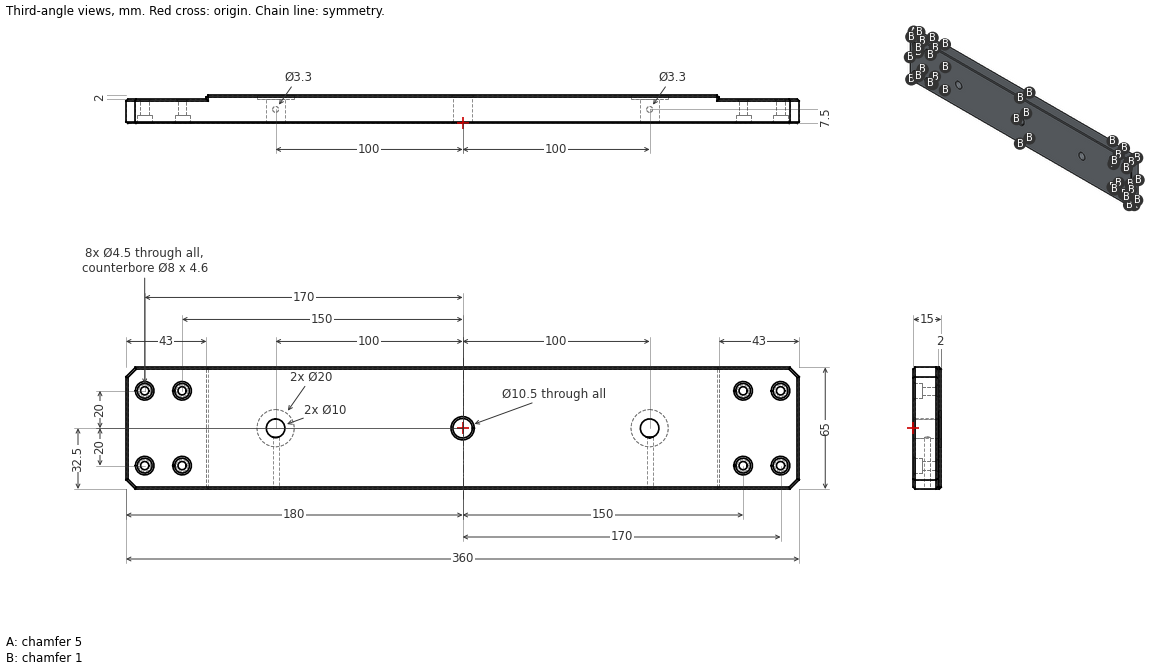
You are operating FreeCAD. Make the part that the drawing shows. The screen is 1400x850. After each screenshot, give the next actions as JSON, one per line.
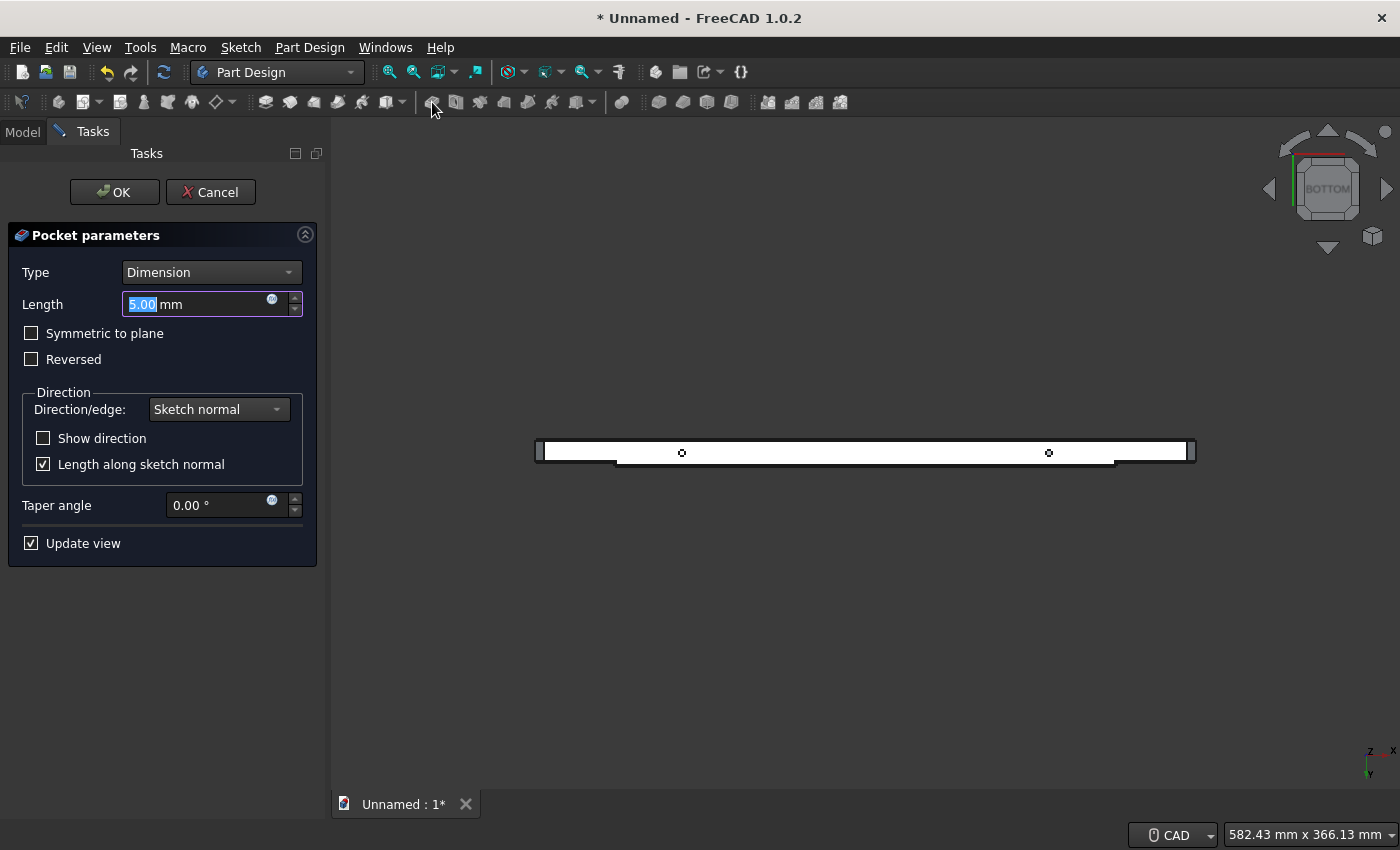
{"action": "left_click", "coordinate": [212, 272]}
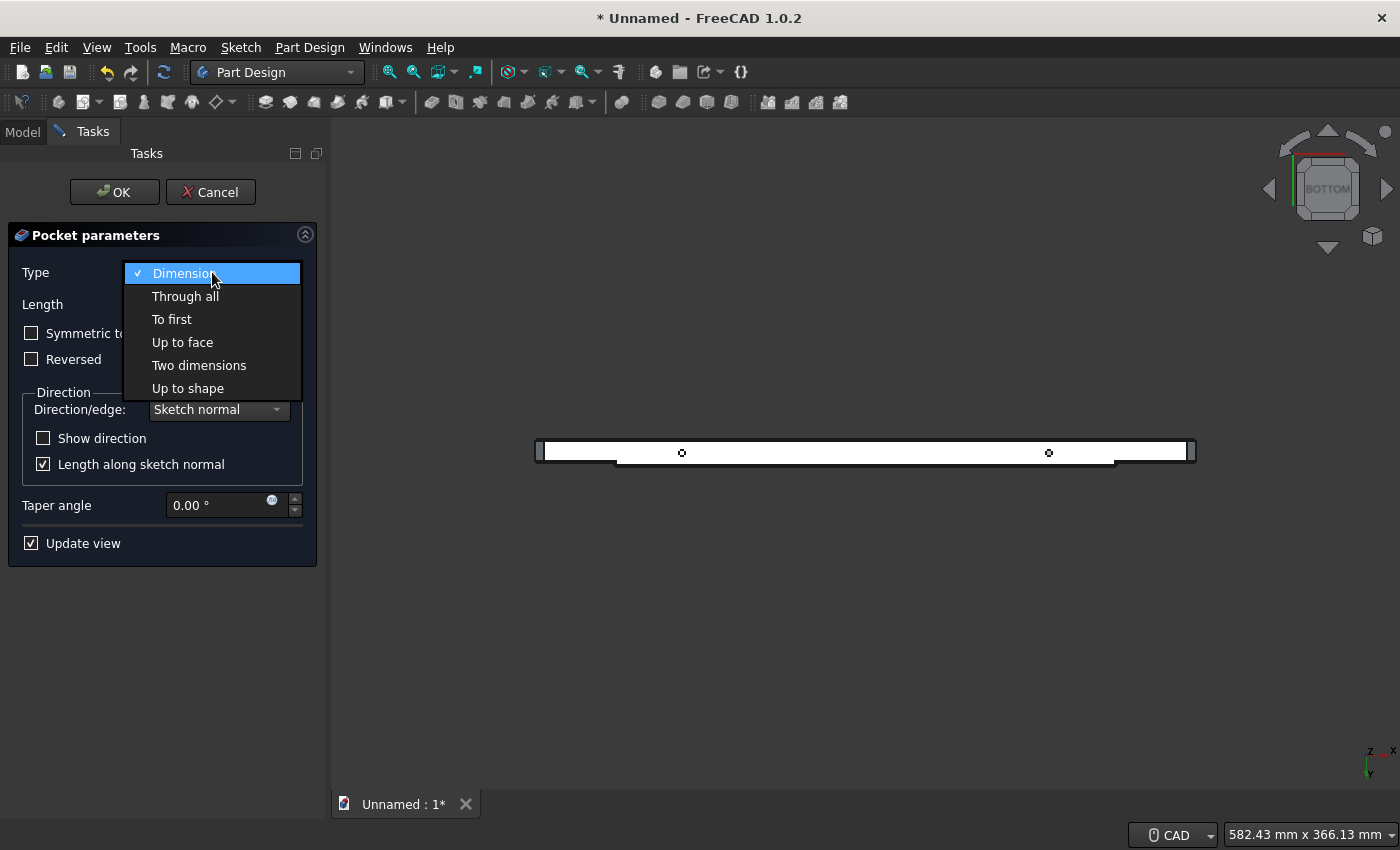
{"action": "left_click", "coordinate": [212, 320]}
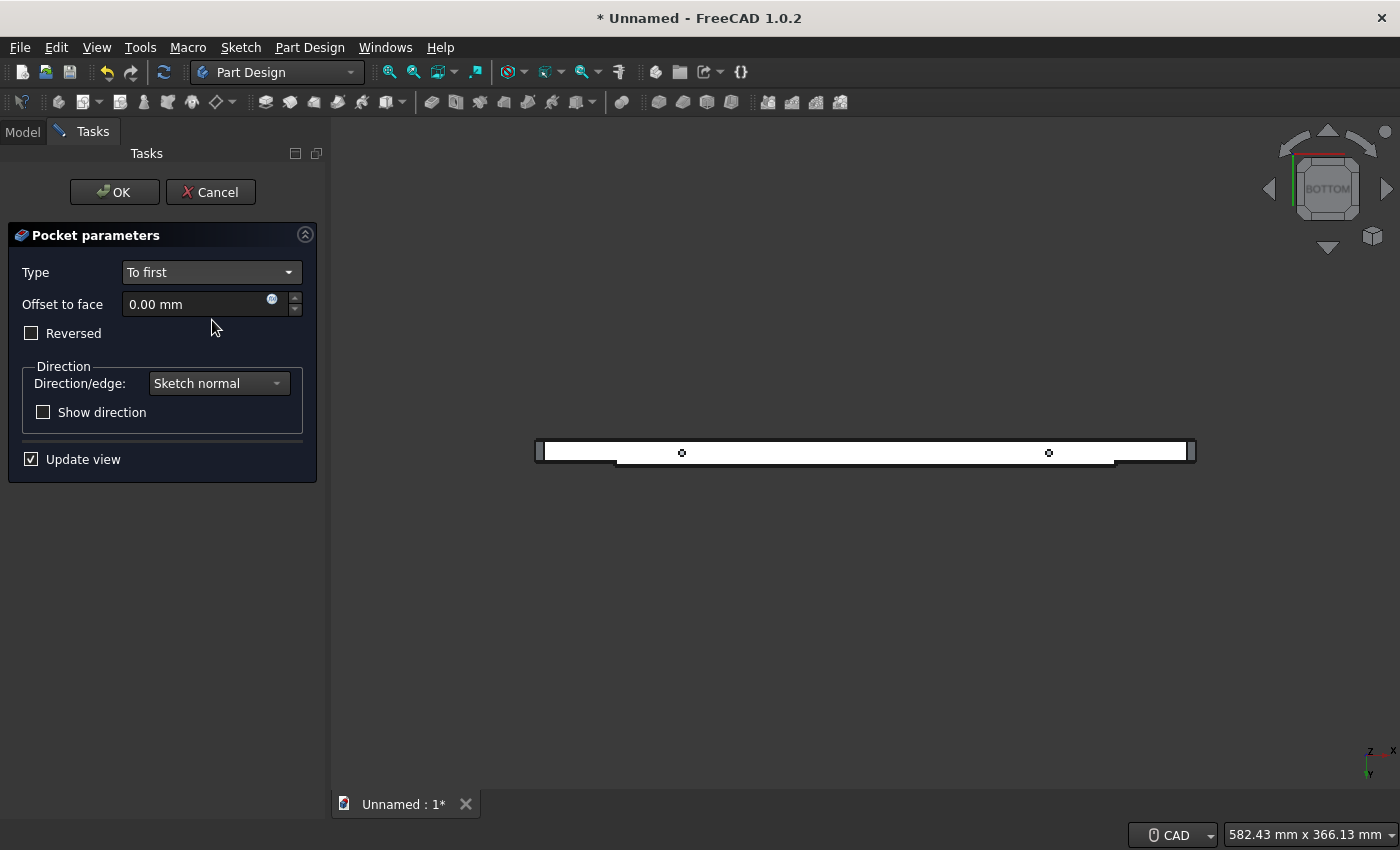
{"action": "left_click", "coordinate": [115, 192]}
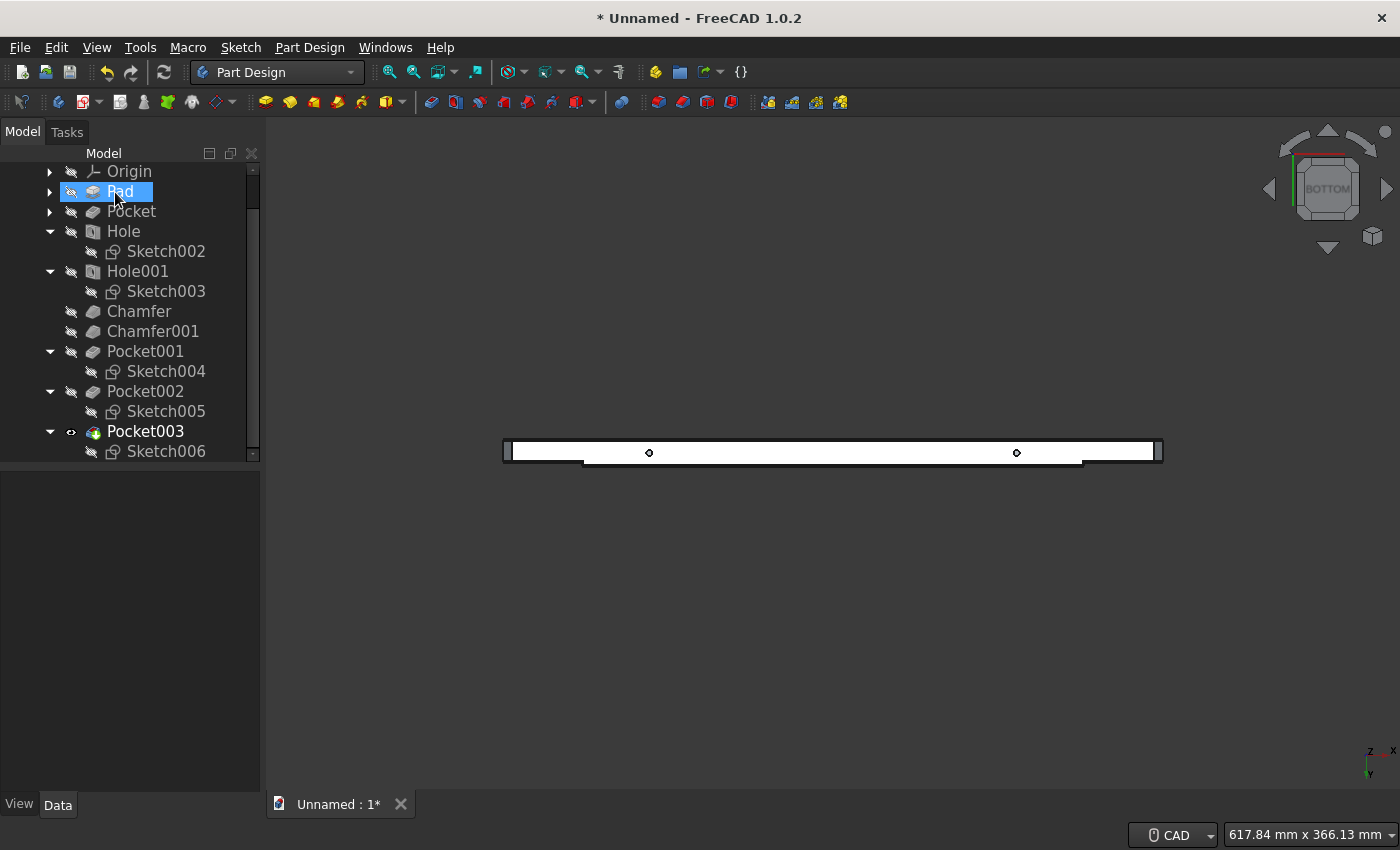
{"action": "key", "text": "4"}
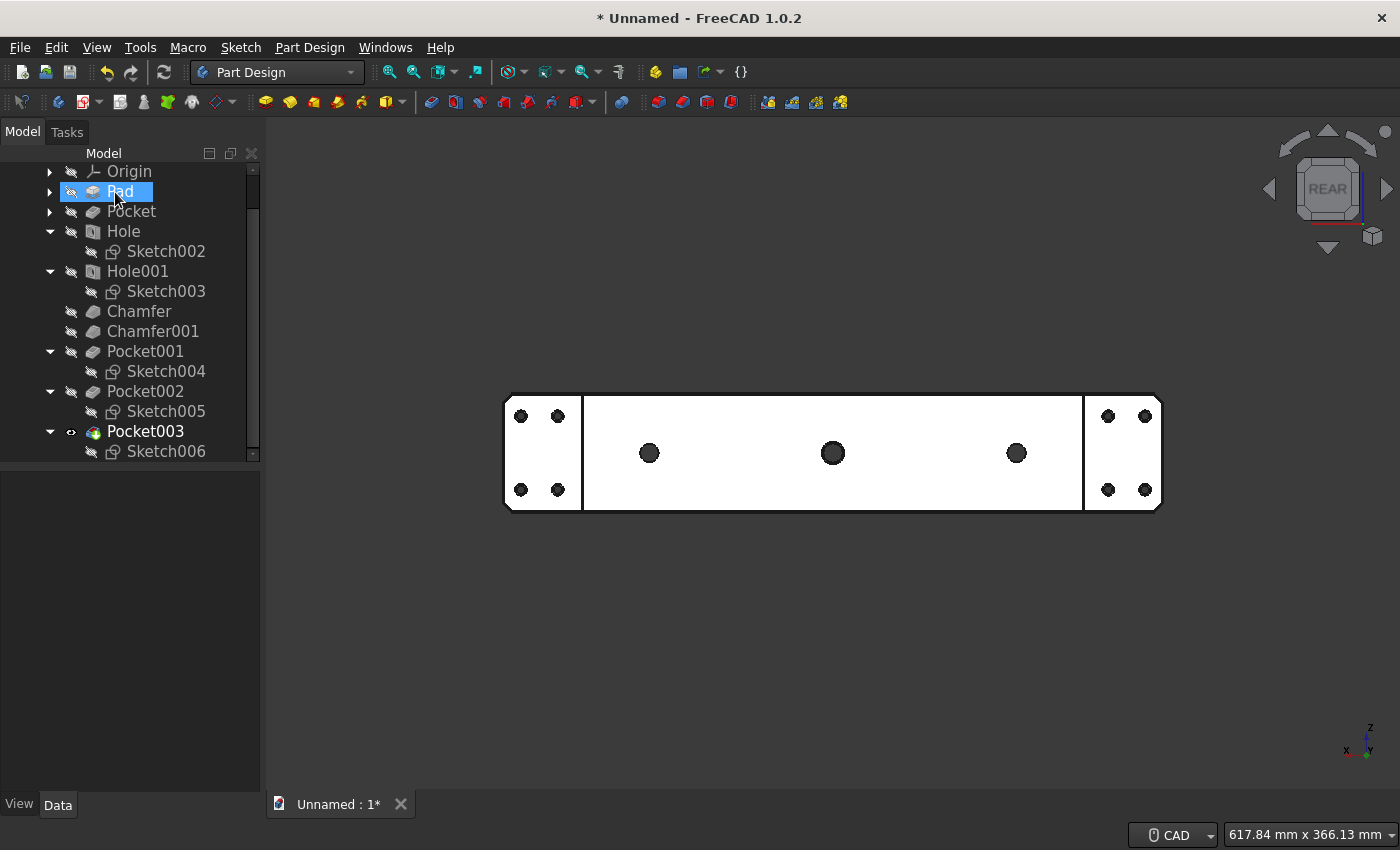
{"action": "left_click", "coordinate": [762, 452]}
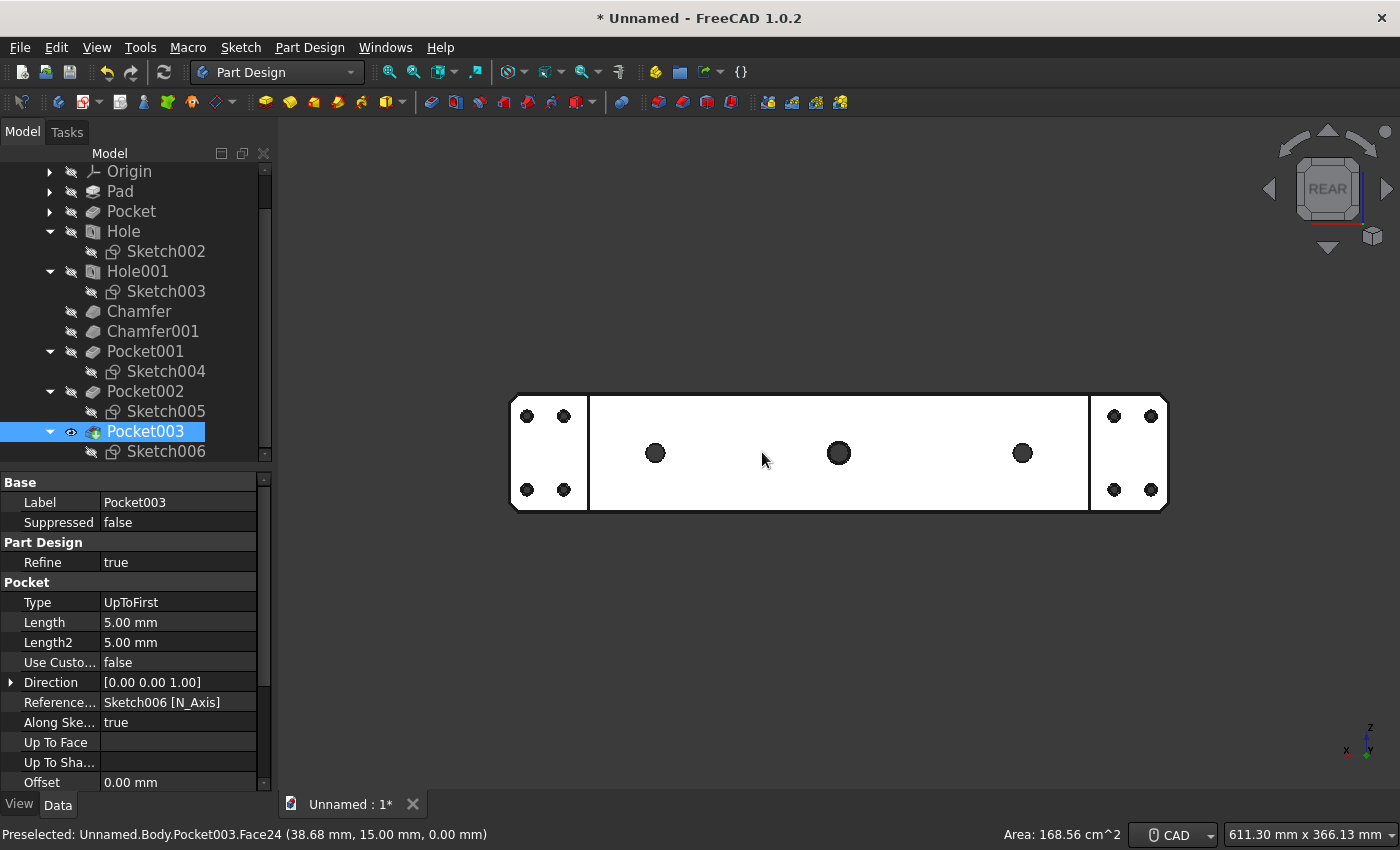
{"action": "left_click", "coordinate": [84, 102]}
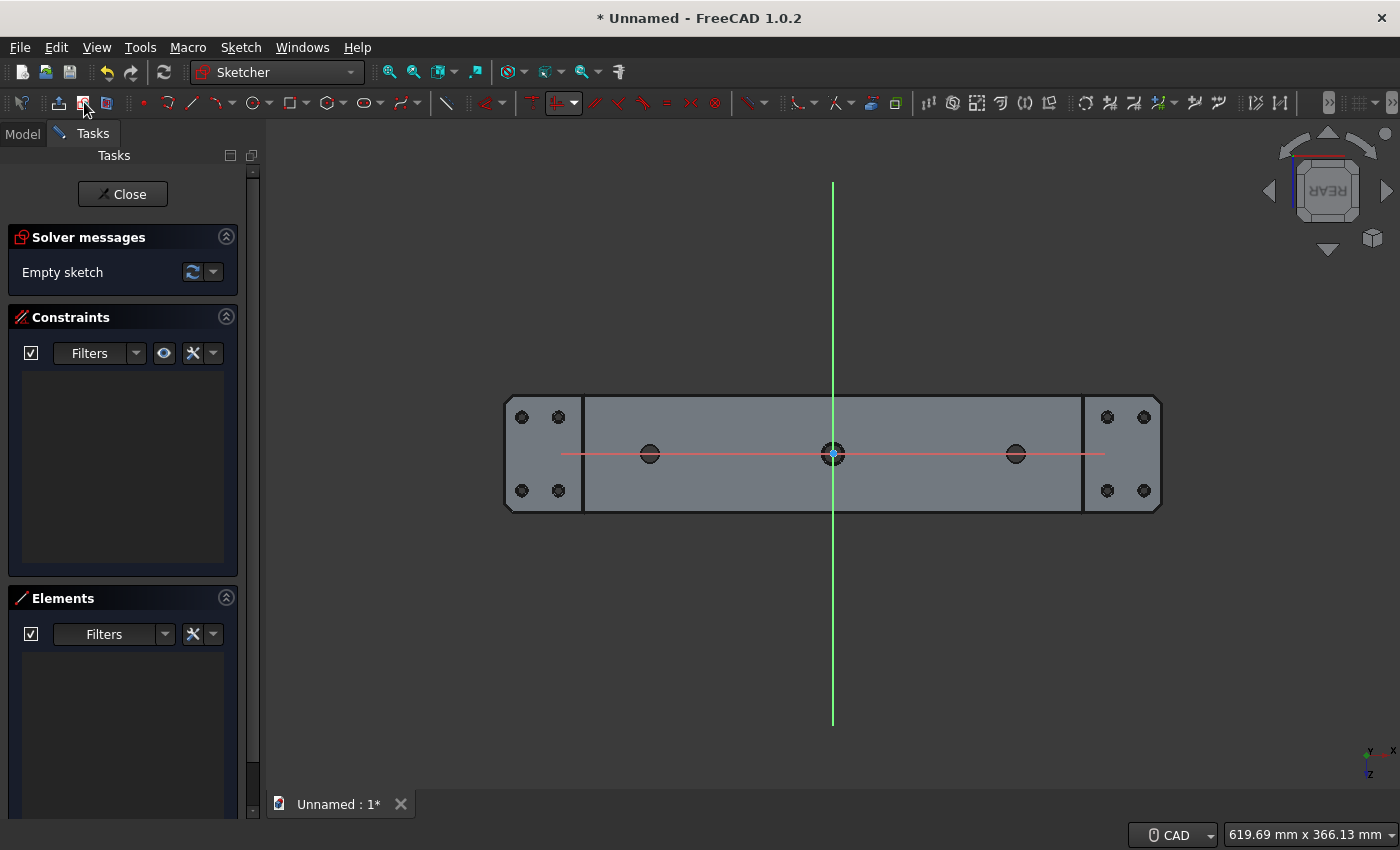
{"action": "scroll", "coordinate": [916, 454], "scroll_direction": "up", "scroll_amount": 3}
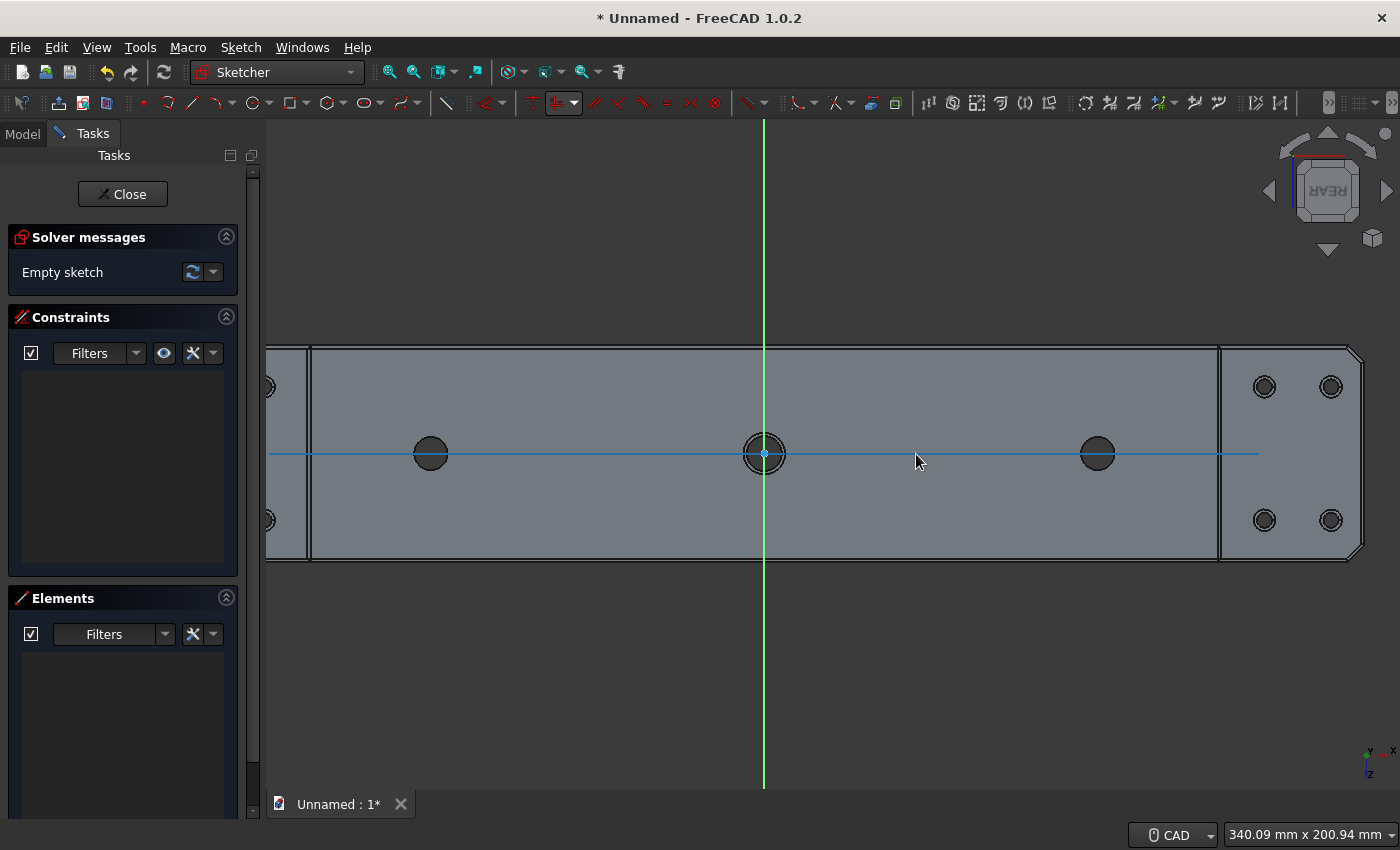
{"action": "key", "text": "g c"}